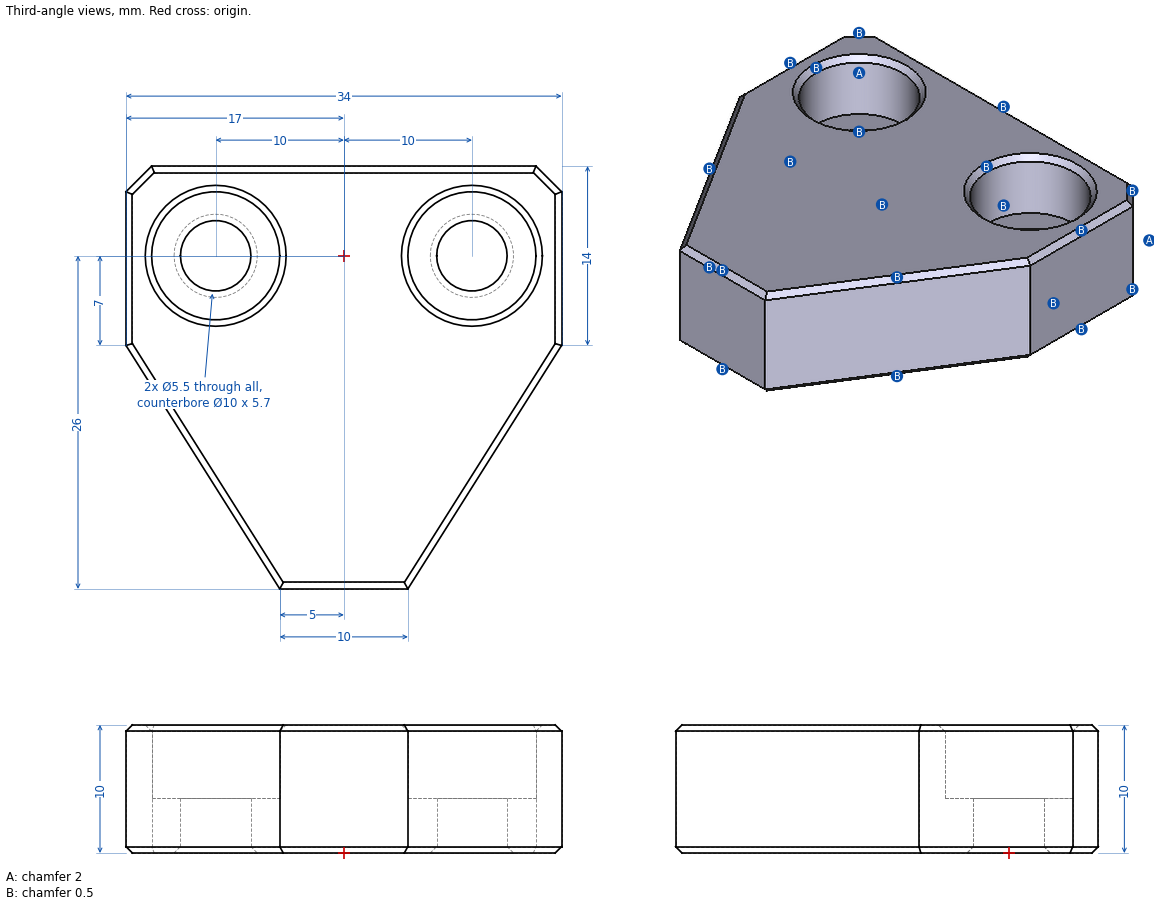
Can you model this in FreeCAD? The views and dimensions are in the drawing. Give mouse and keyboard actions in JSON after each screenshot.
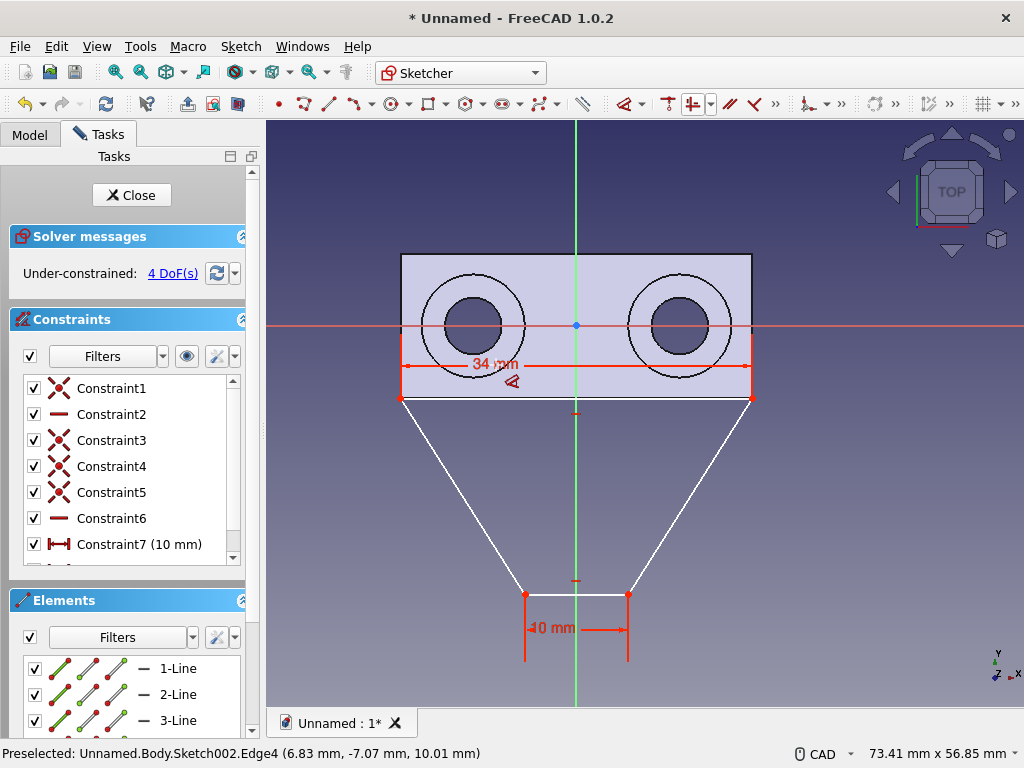
{"action": "left_click", "coordinate": [401, 399]}
{"action": "left_click", "coordinate": [367, 362]}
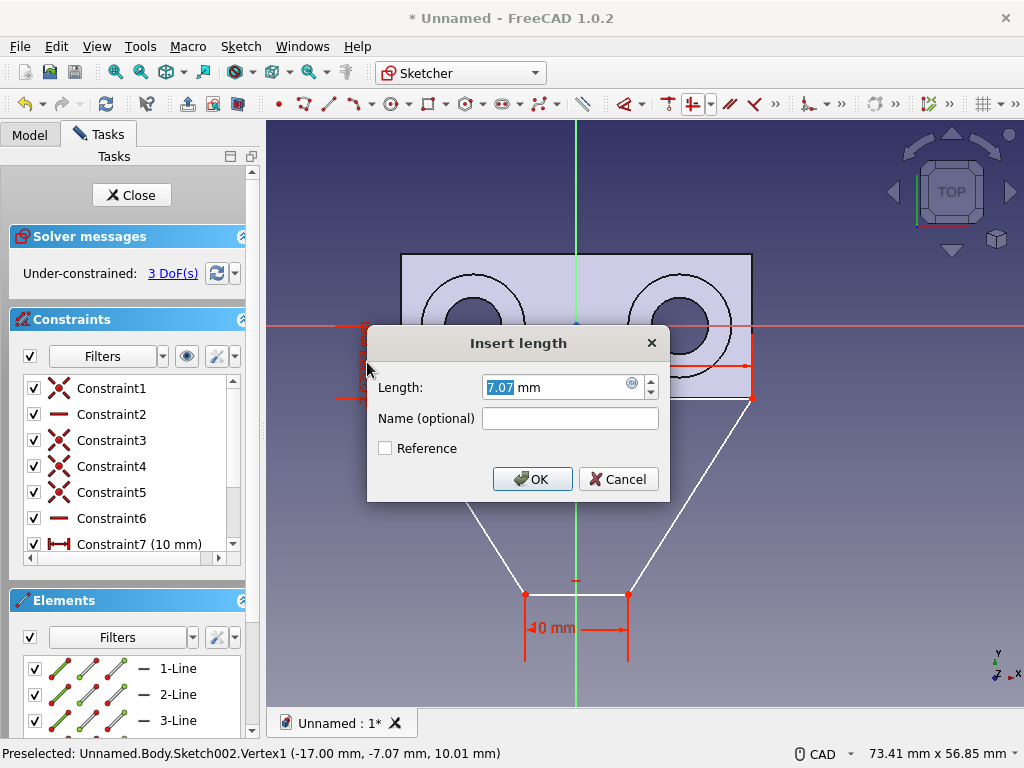
{"action": "type", "text": "7"}
{"action": "key", "text": "Return"}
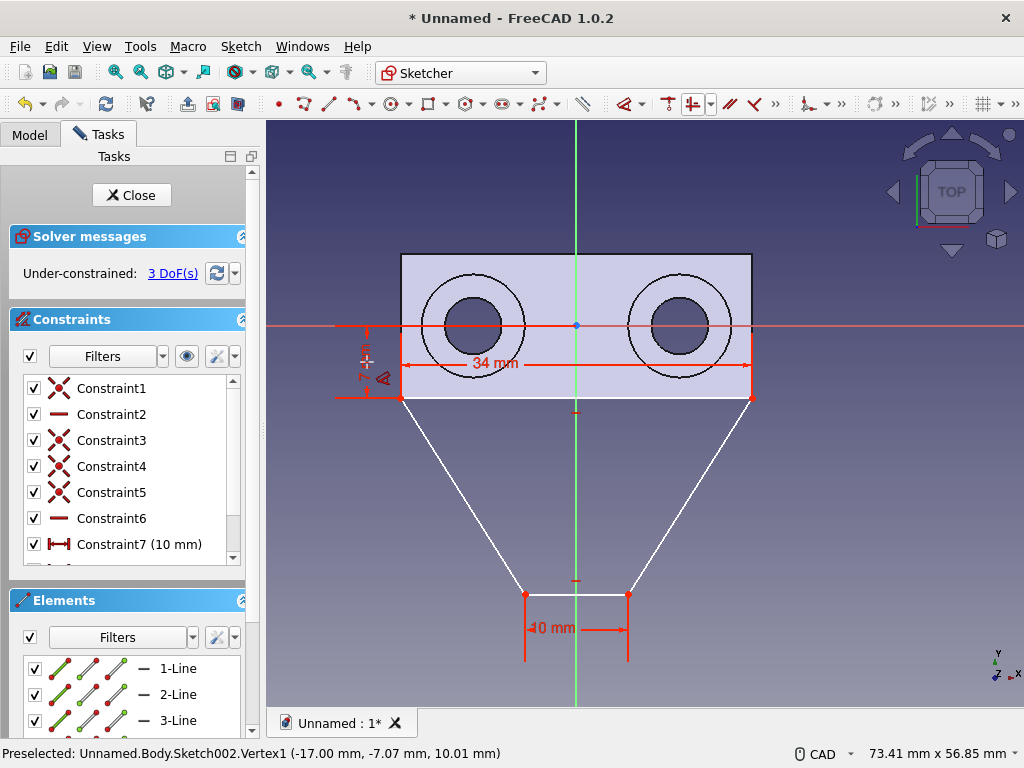
{"action": "left_click", "coordinate": [525, 595]}
{"action": "left_click", "coordinate": [551, 292]}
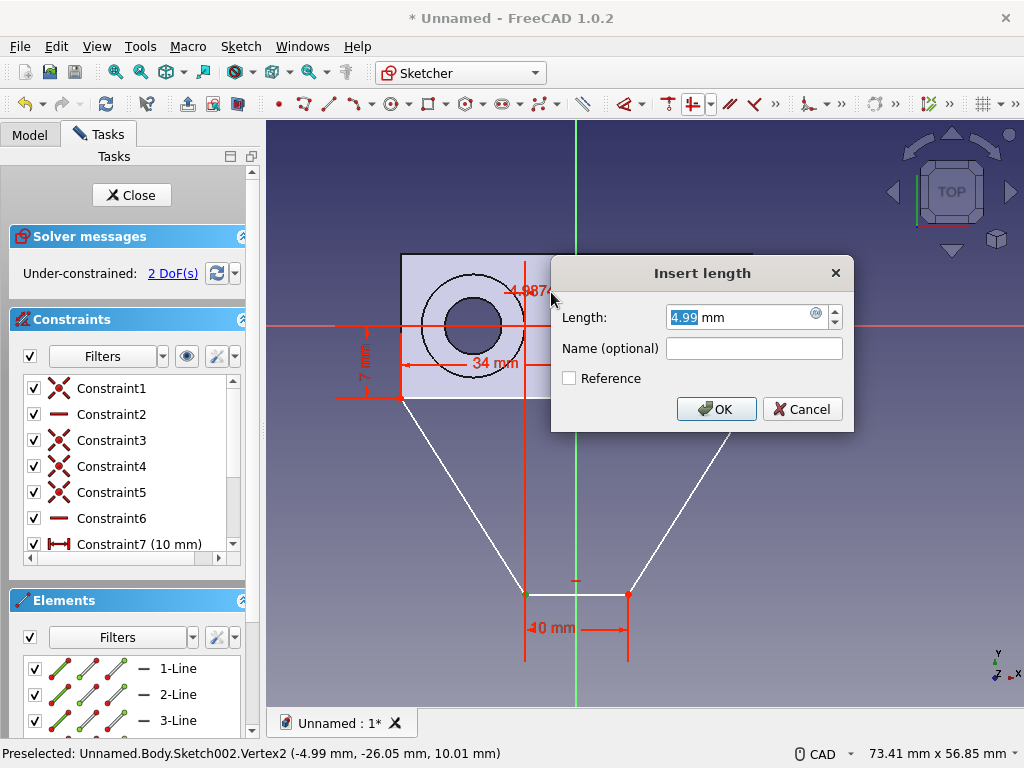
{"action": "type", "text": "5"}
{"action": "key", "text": "Return"}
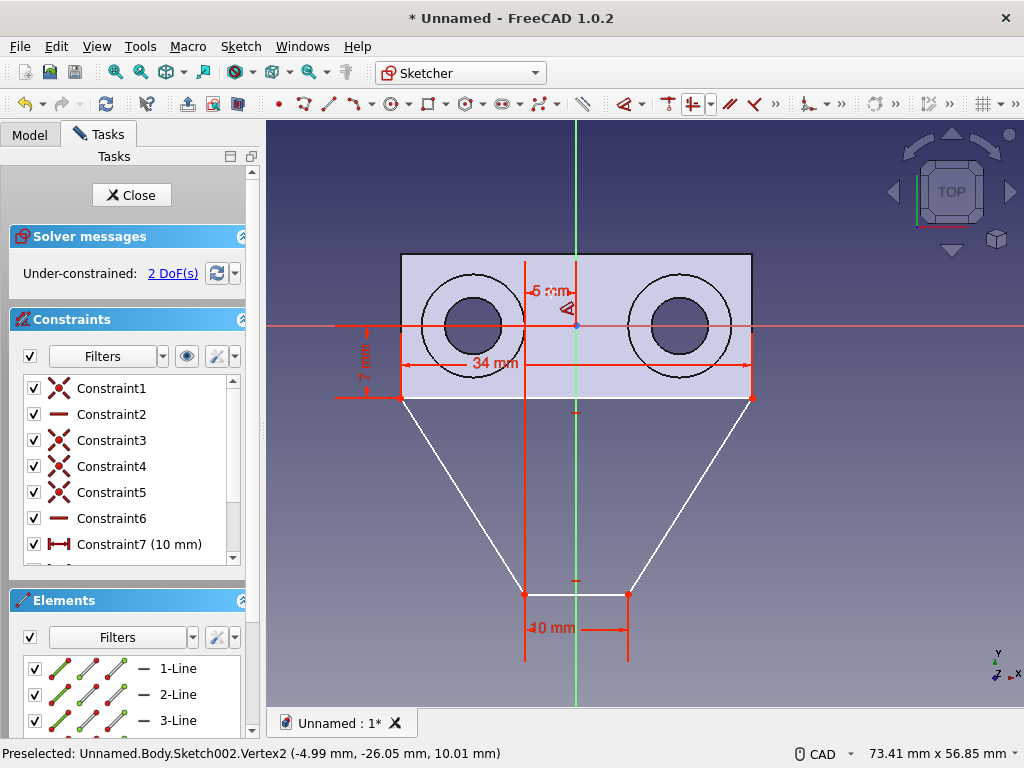
{"action": "left_click", "coordinate": [401, 398]}
{"action": "left_click", "coordinate": [448, 292]}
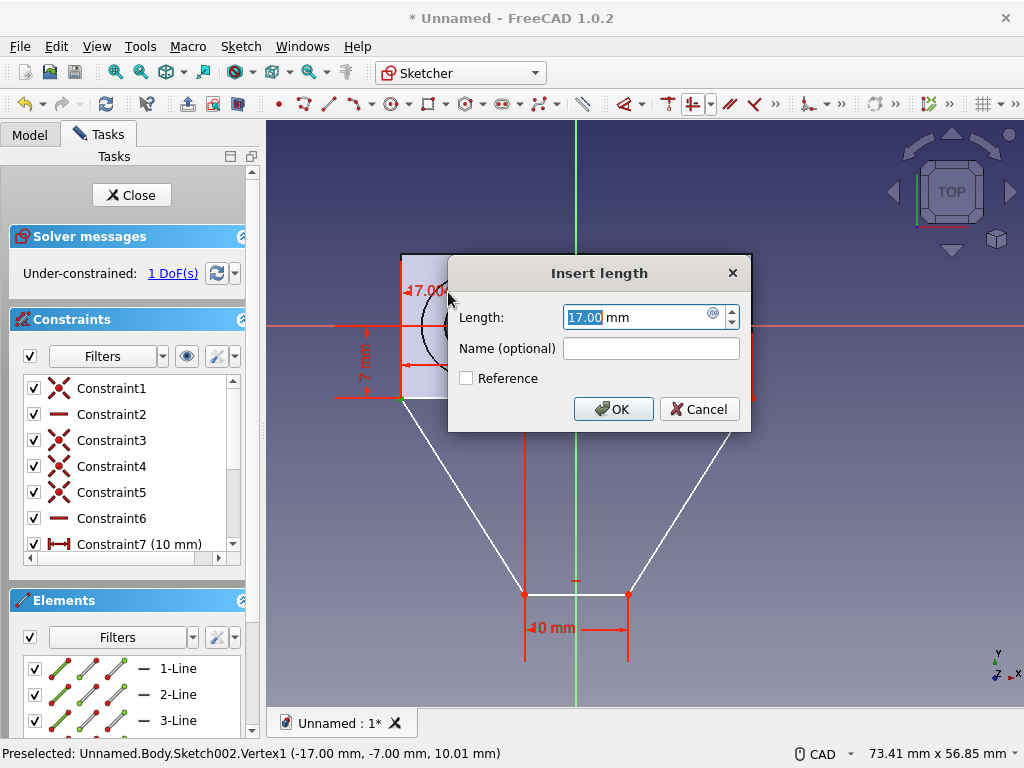
{"action": "type", "text": "17"}
{"action": "key", "text": "Return"}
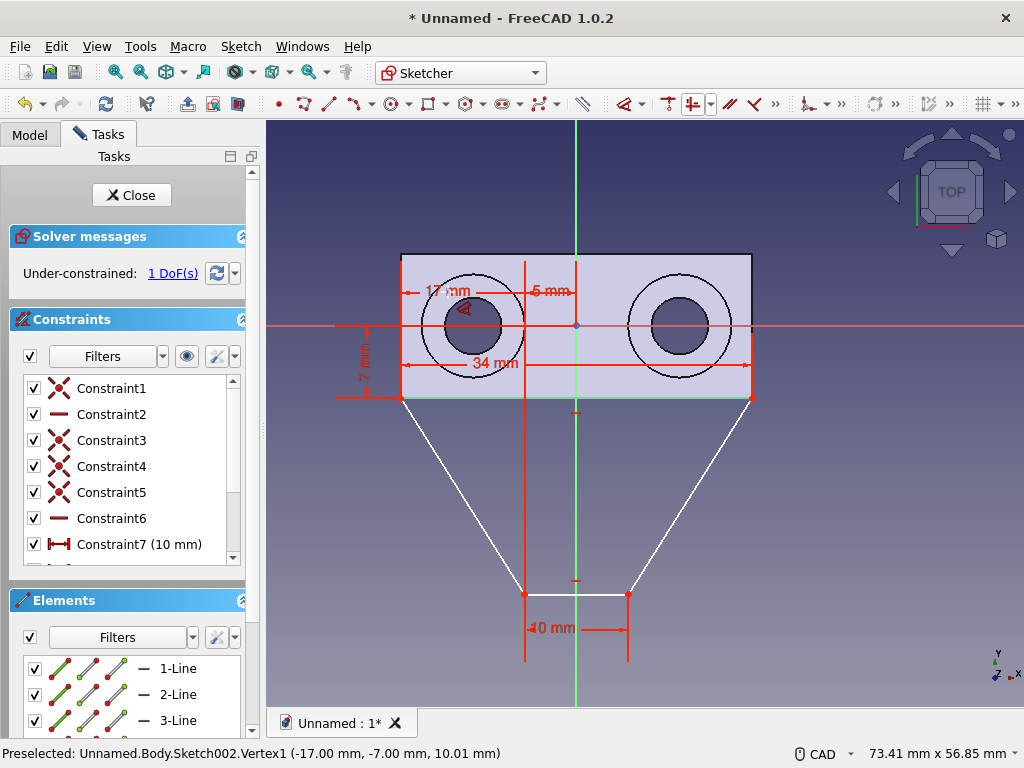
{"action": "left_click", "coordinate": [525, 595]}
{"action": "left_click", "coordinate": [491, 460]}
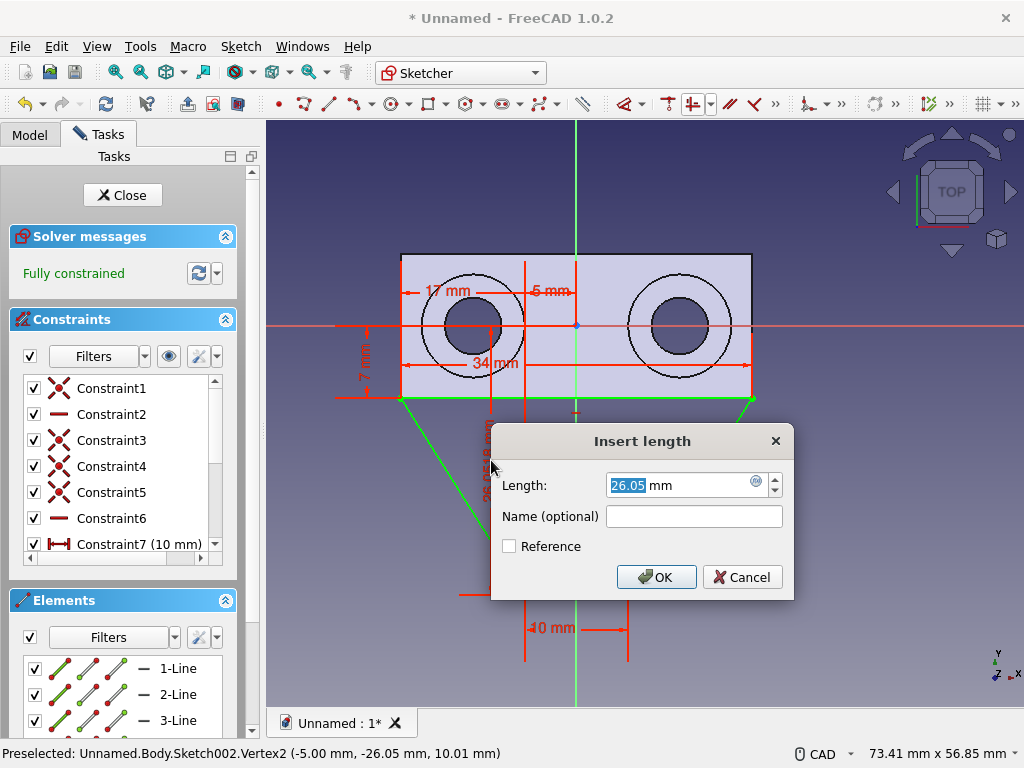
{"action": "type", "text": "26"}
{"action": "key", "text": "Return"}
{"action": "key", "text": "Escape"}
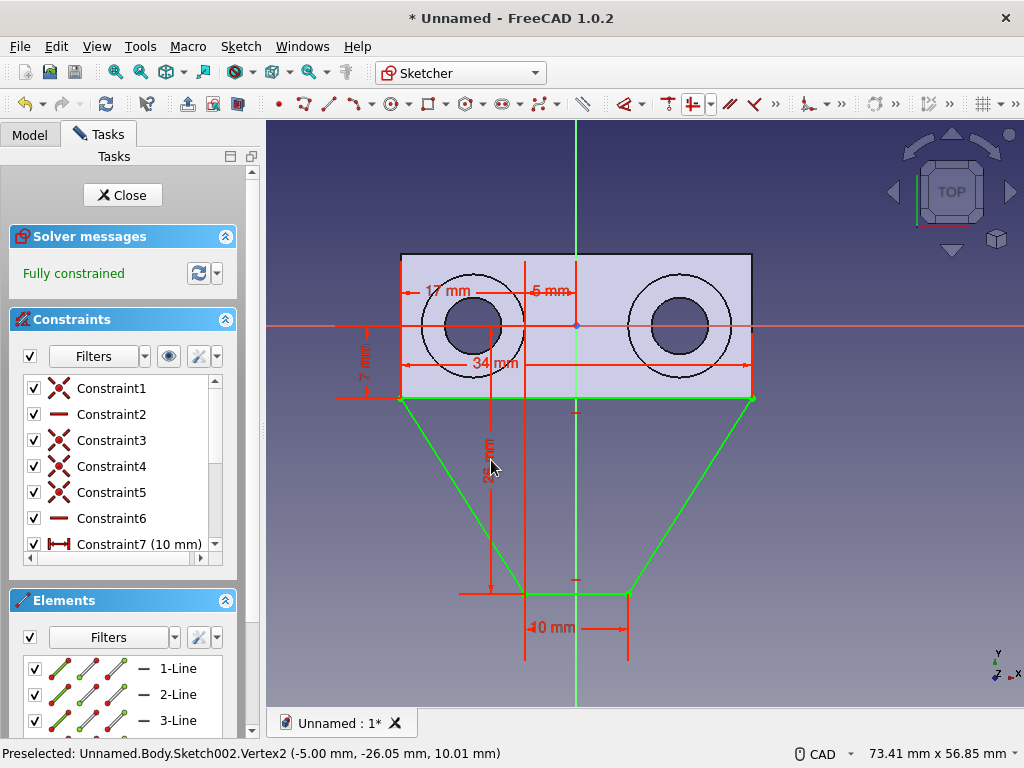
{"action": "left_click", "coordinate": [123, 195]}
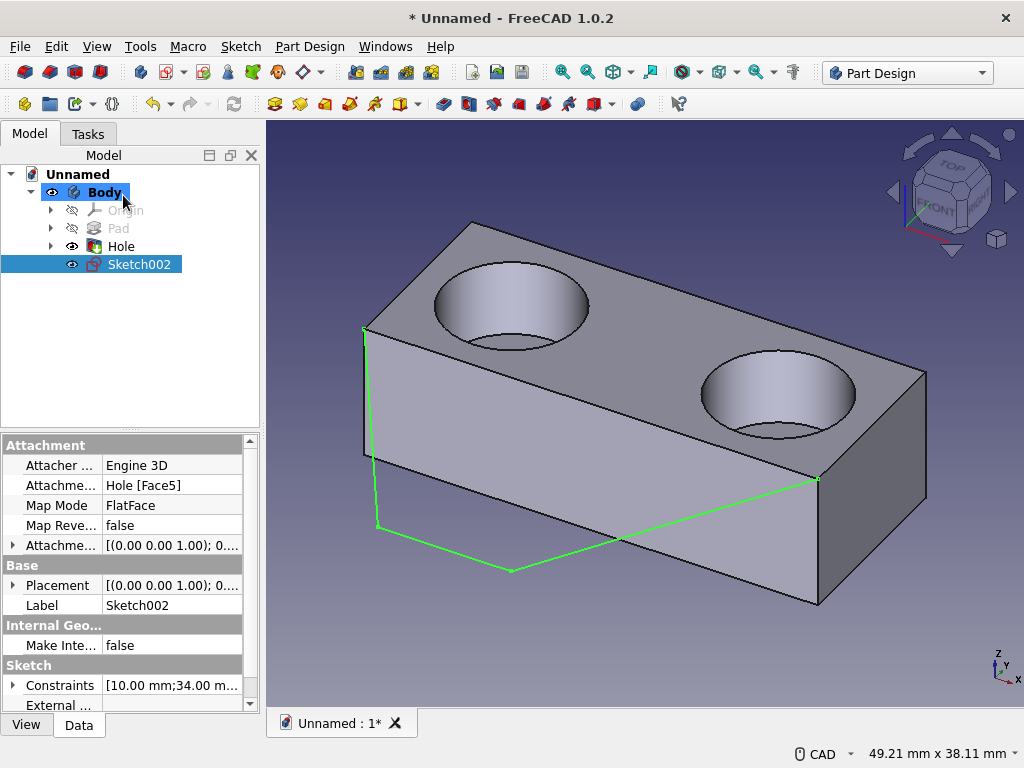
{"action": "left_click", "coordinate": [275, 104]}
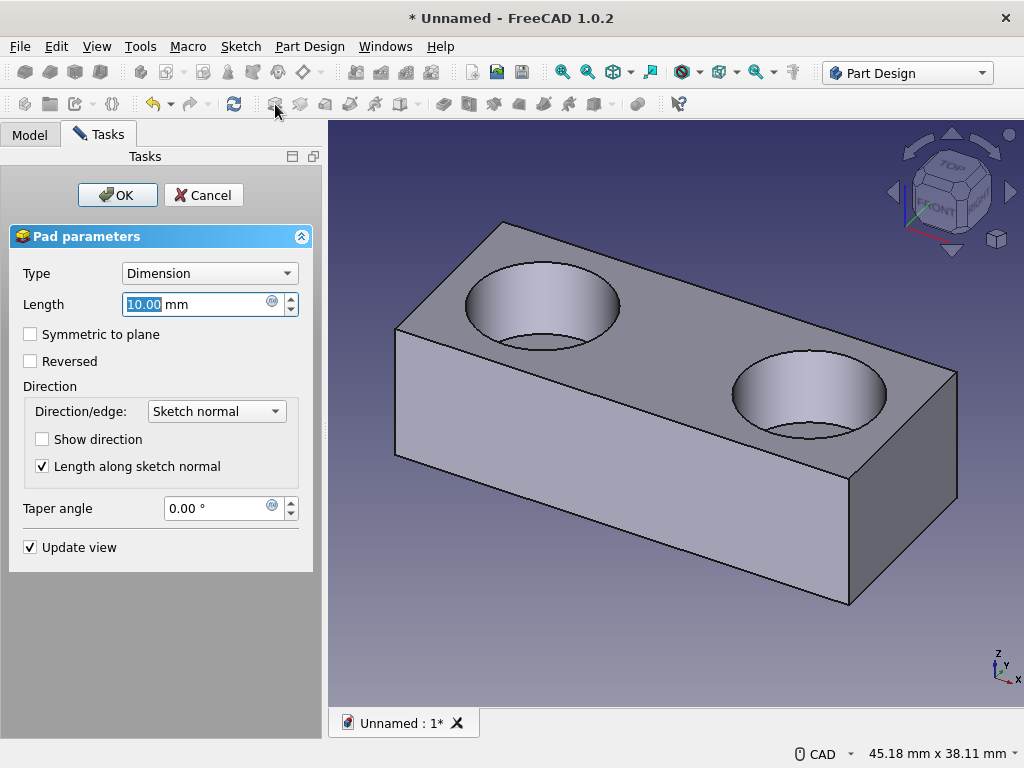
{"action": "type", "text": "10"}
{"action": "key", "text": "Tab"}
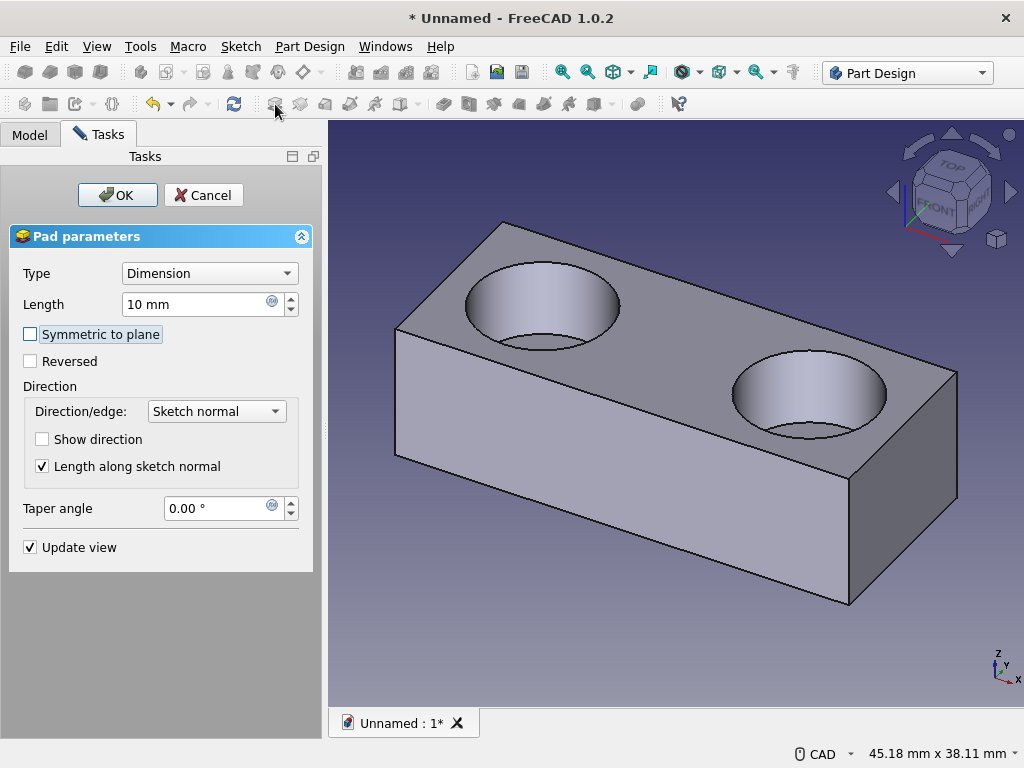
{"action": "left_click", "coordinate": [31, 361]}